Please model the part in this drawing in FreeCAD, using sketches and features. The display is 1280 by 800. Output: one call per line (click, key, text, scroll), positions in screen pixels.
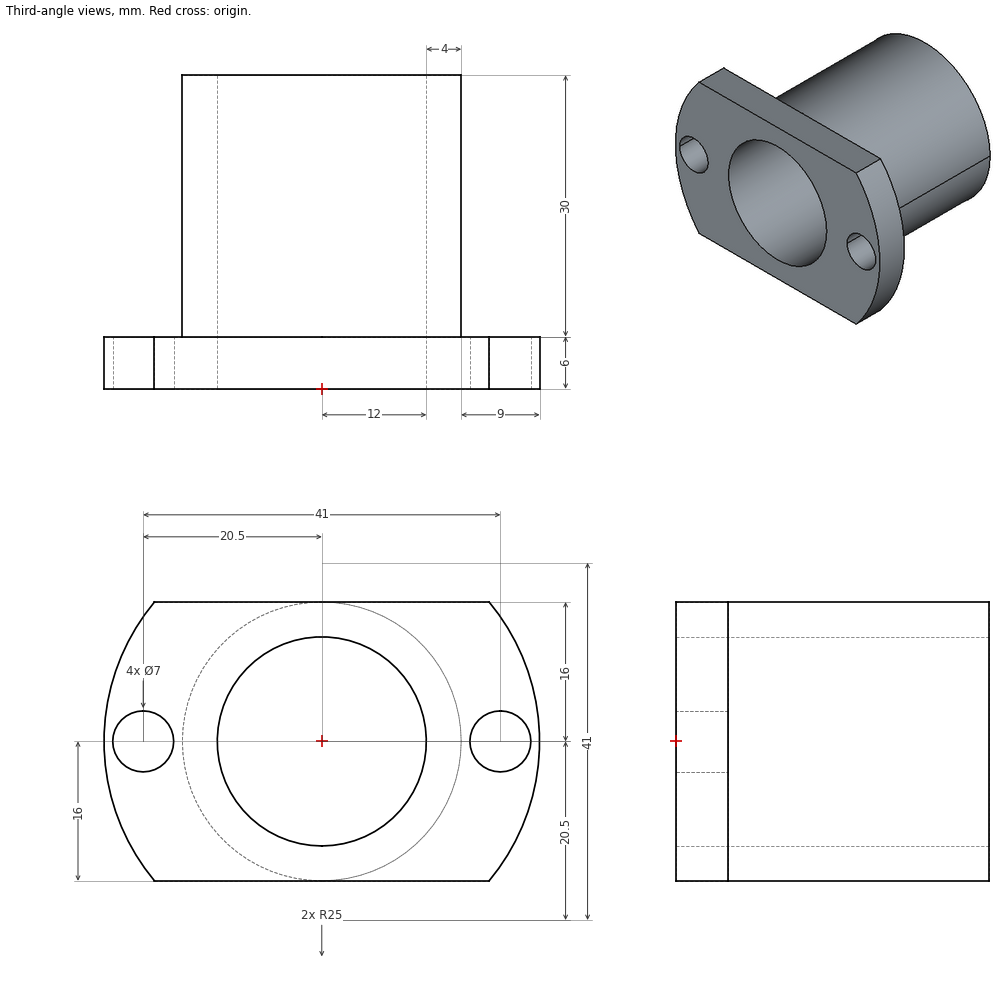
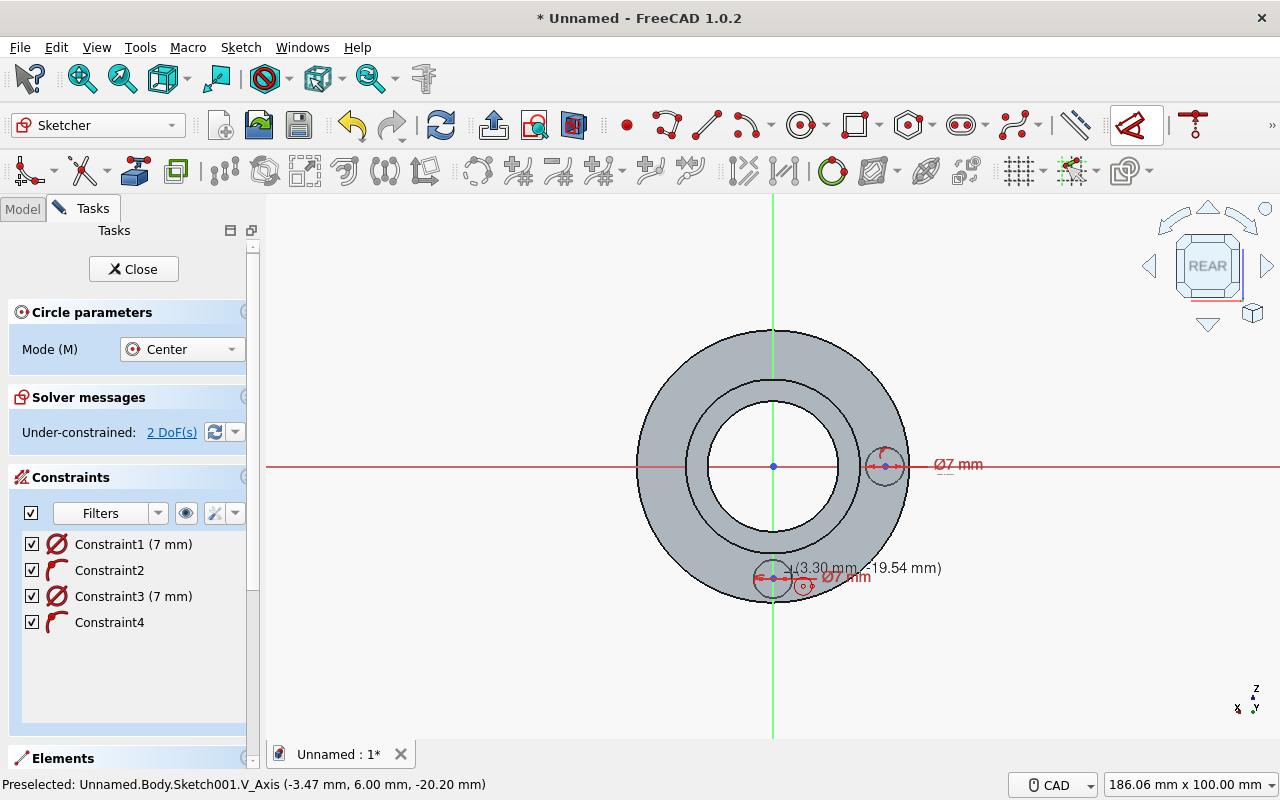
click(661, 466)
move(668, 449)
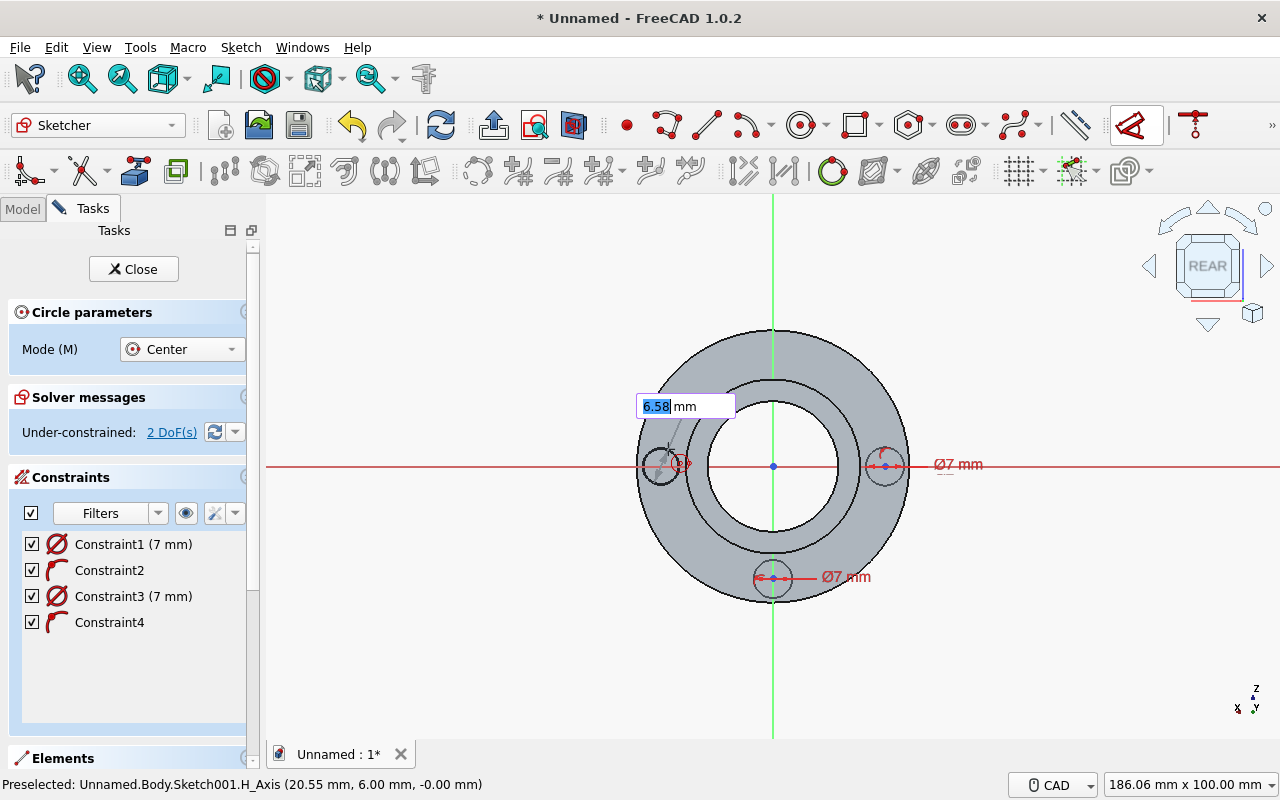
text(7)
key(Return)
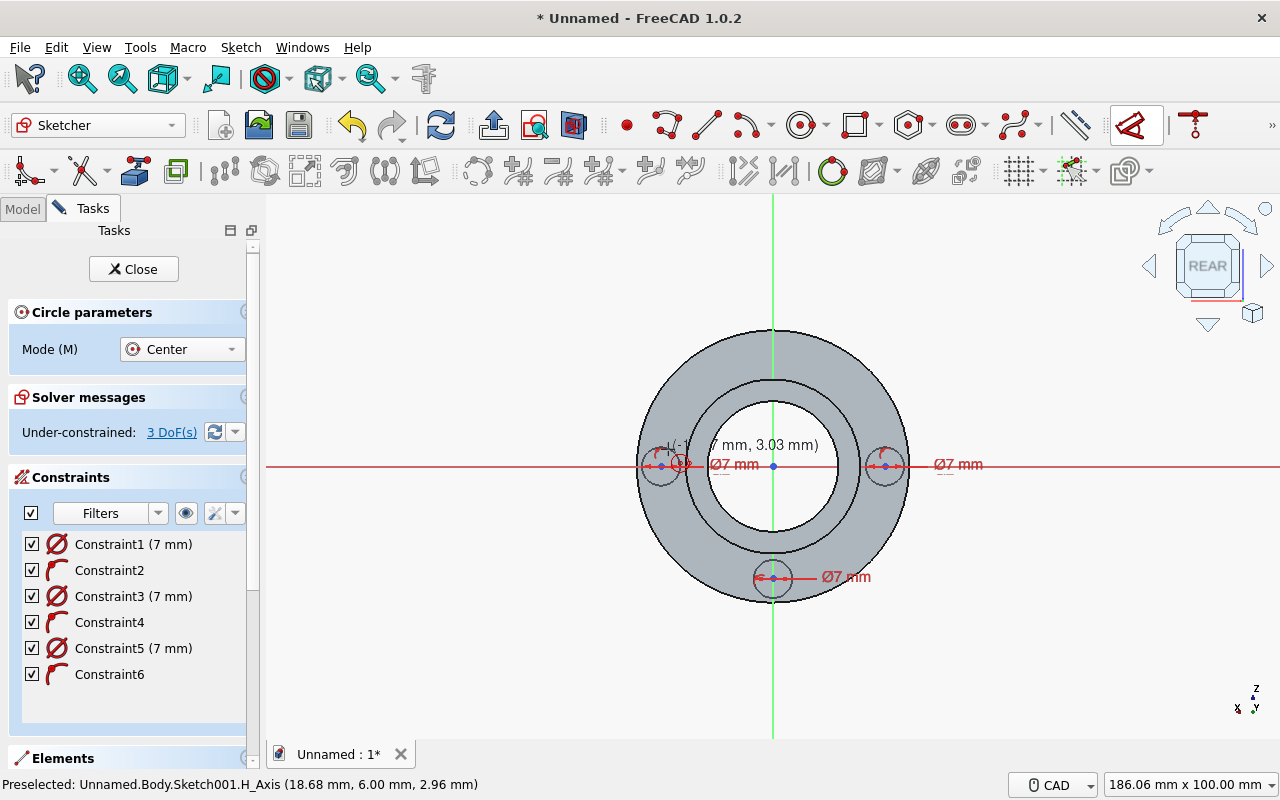
click(773, 355)
move(791, 348)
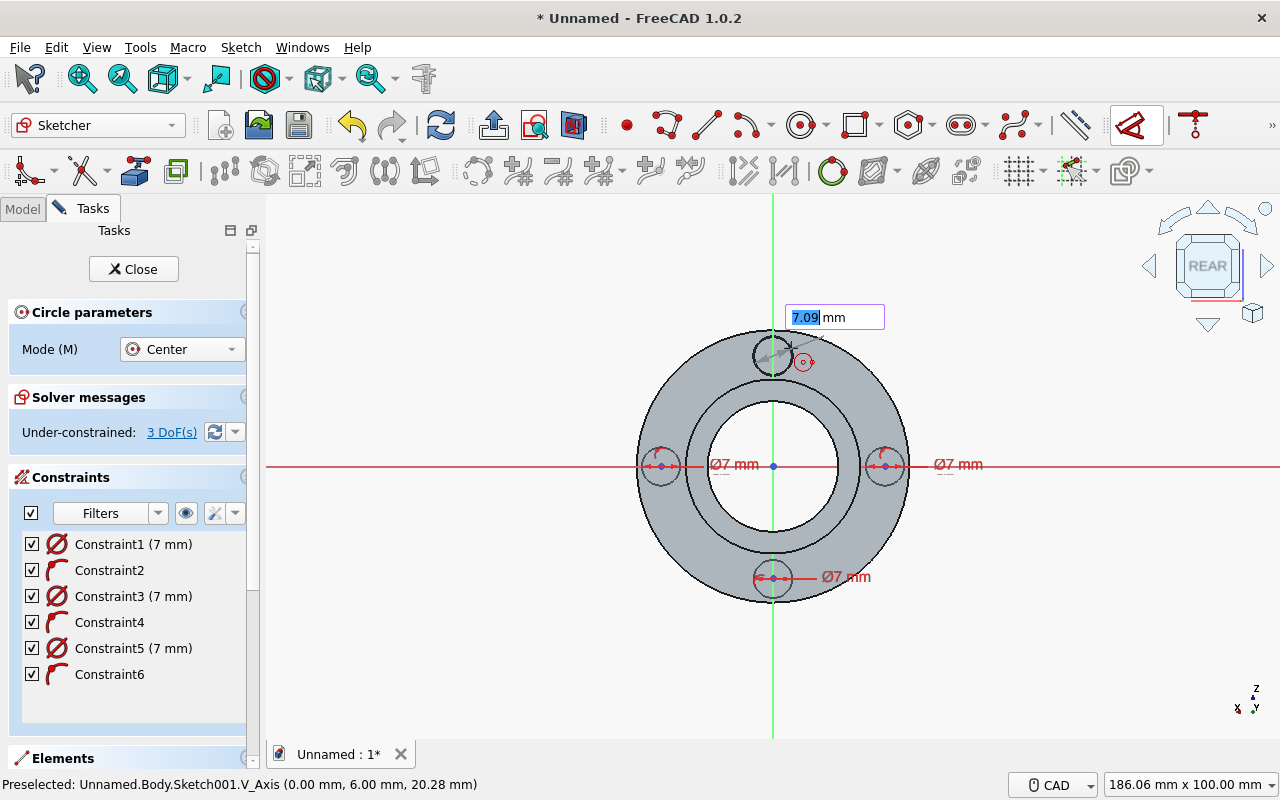
text(7)
key(Return)
key(Escape)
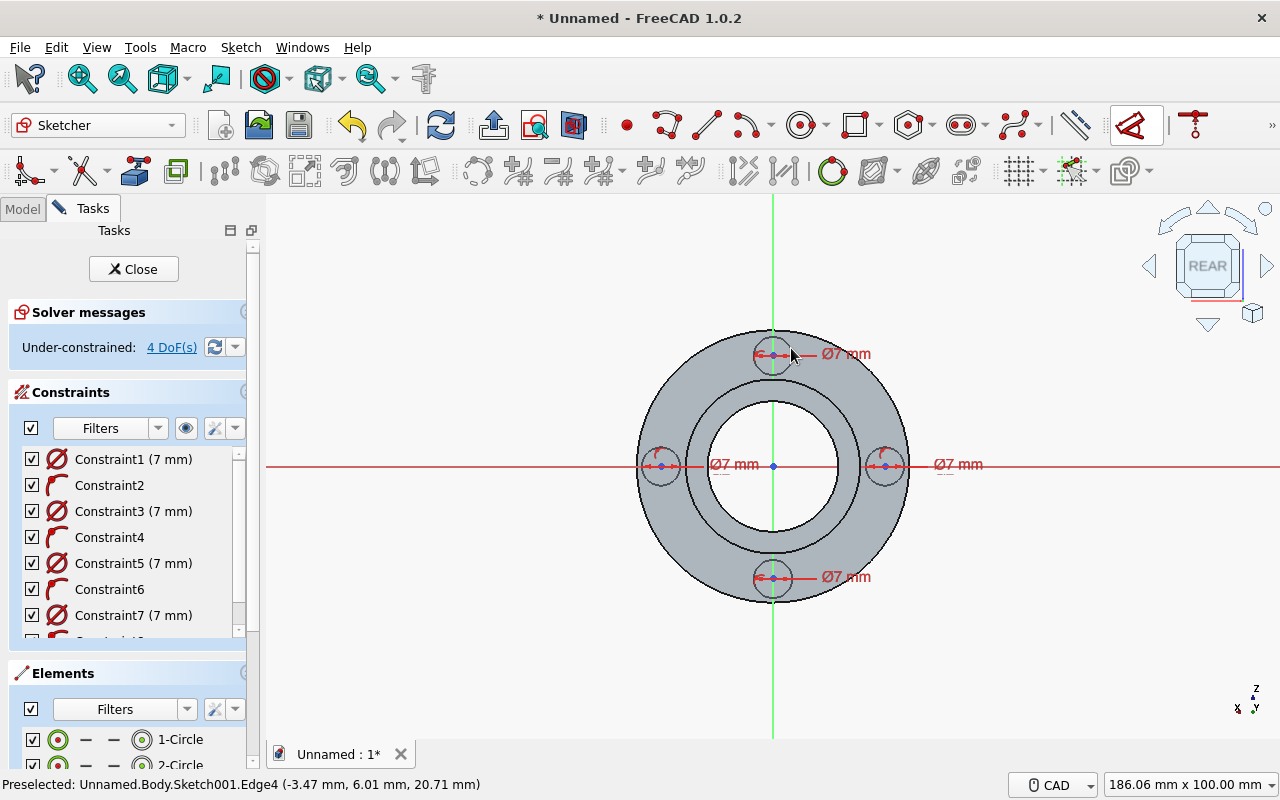
click(885, 466)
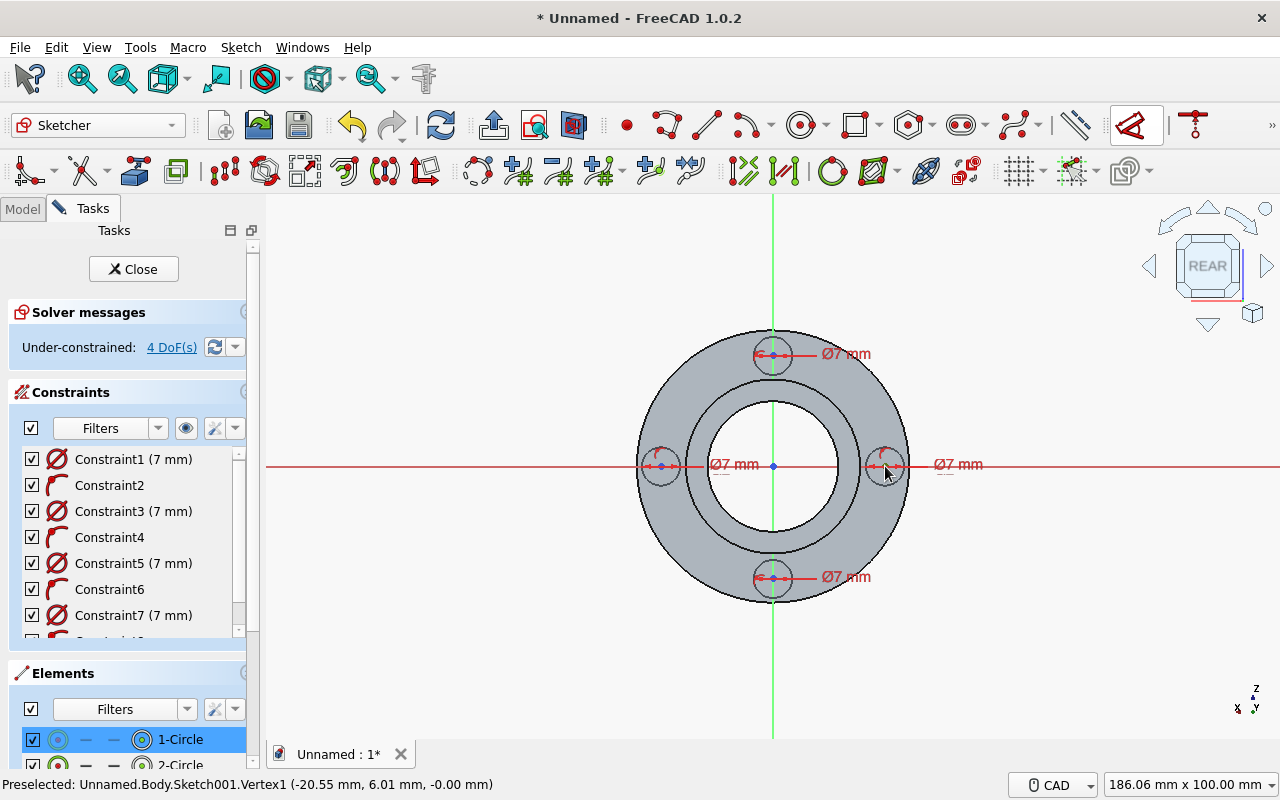
click(661, 466)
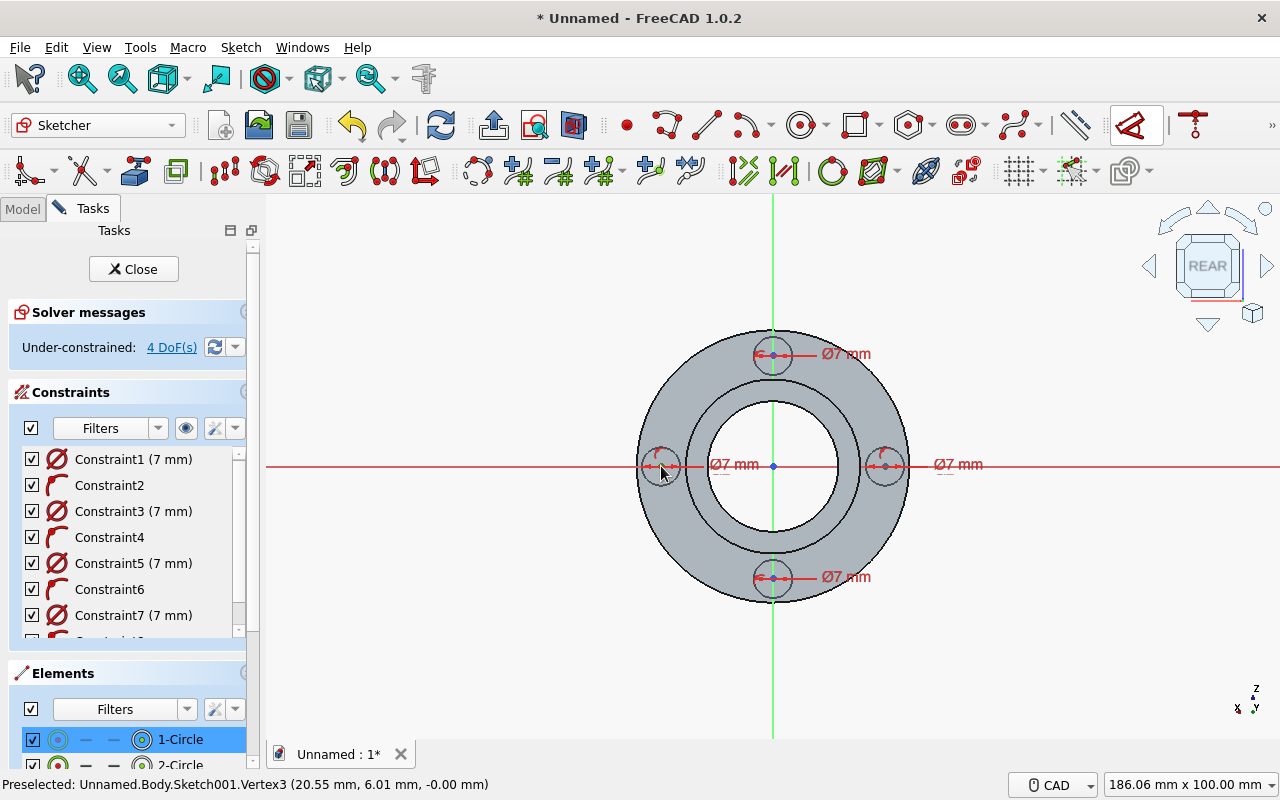
click(1158, 126)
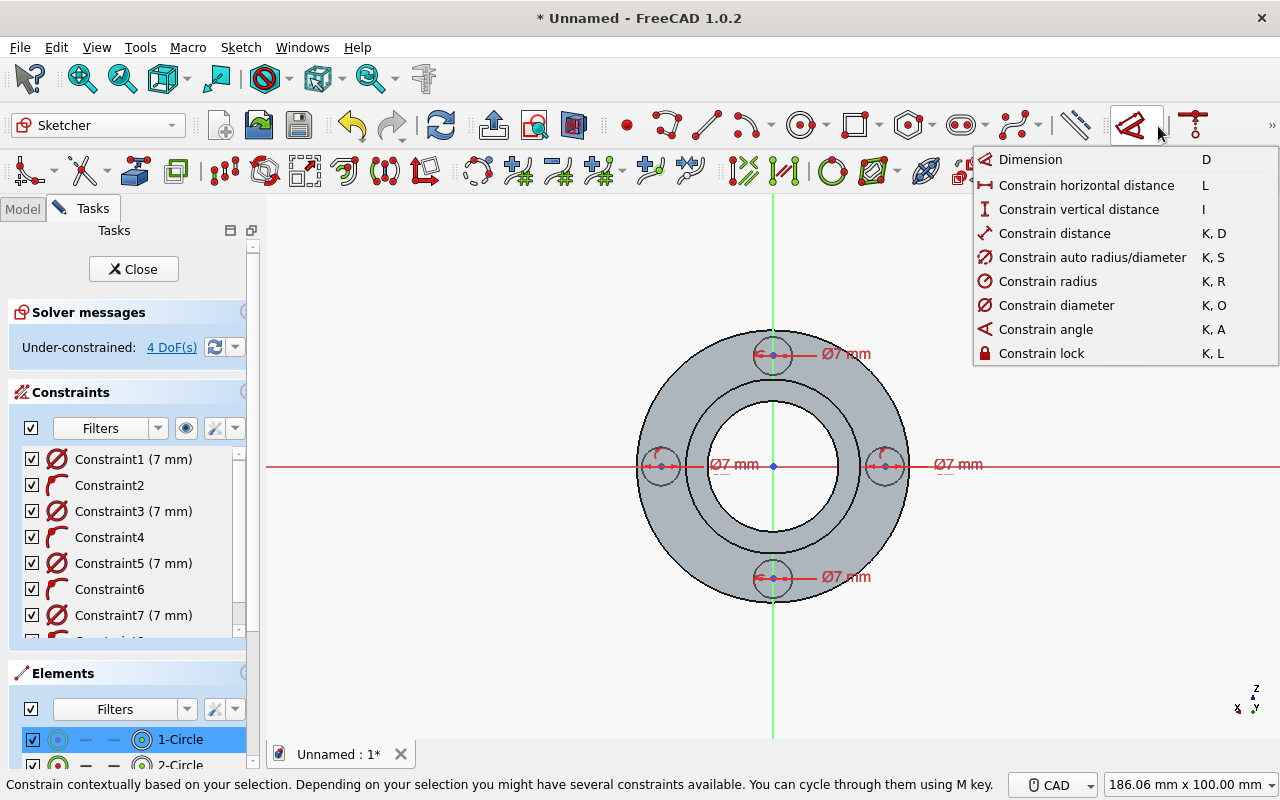
click(1126, 185)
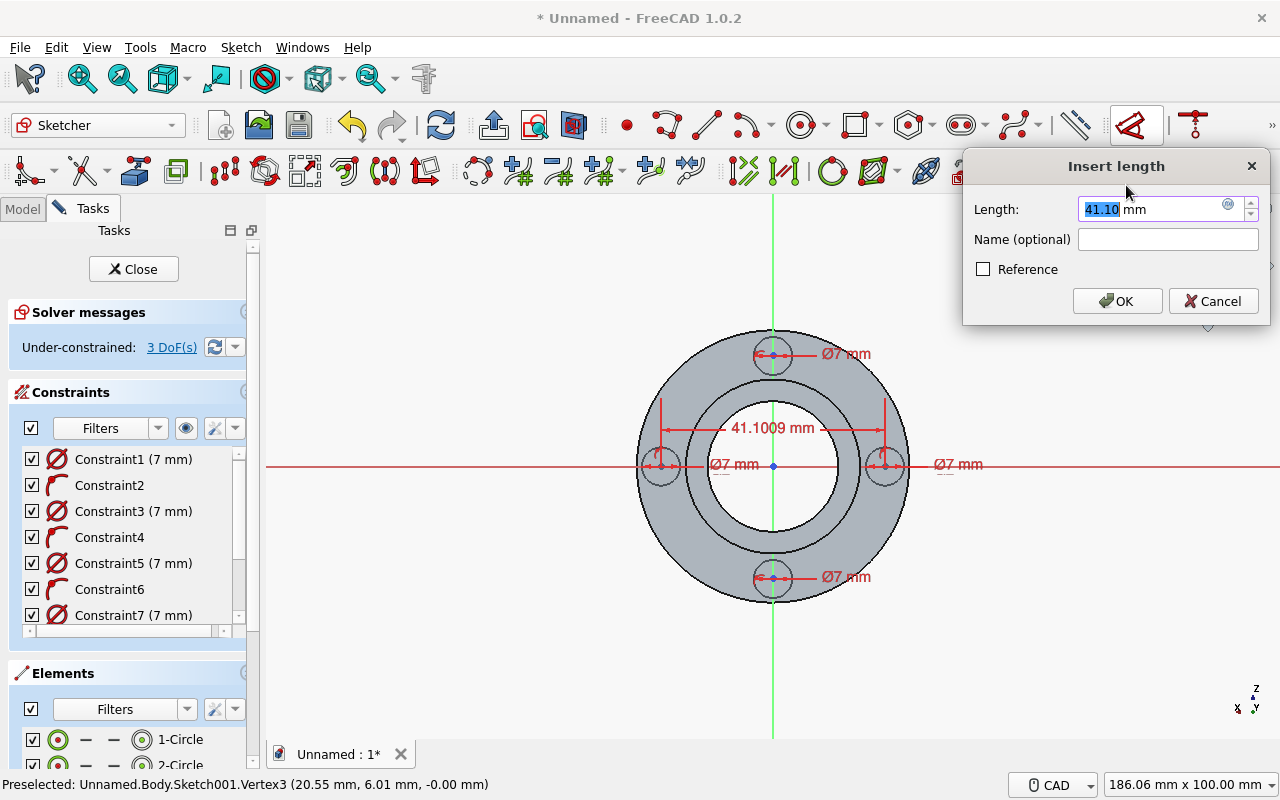
text(41)
key(Return)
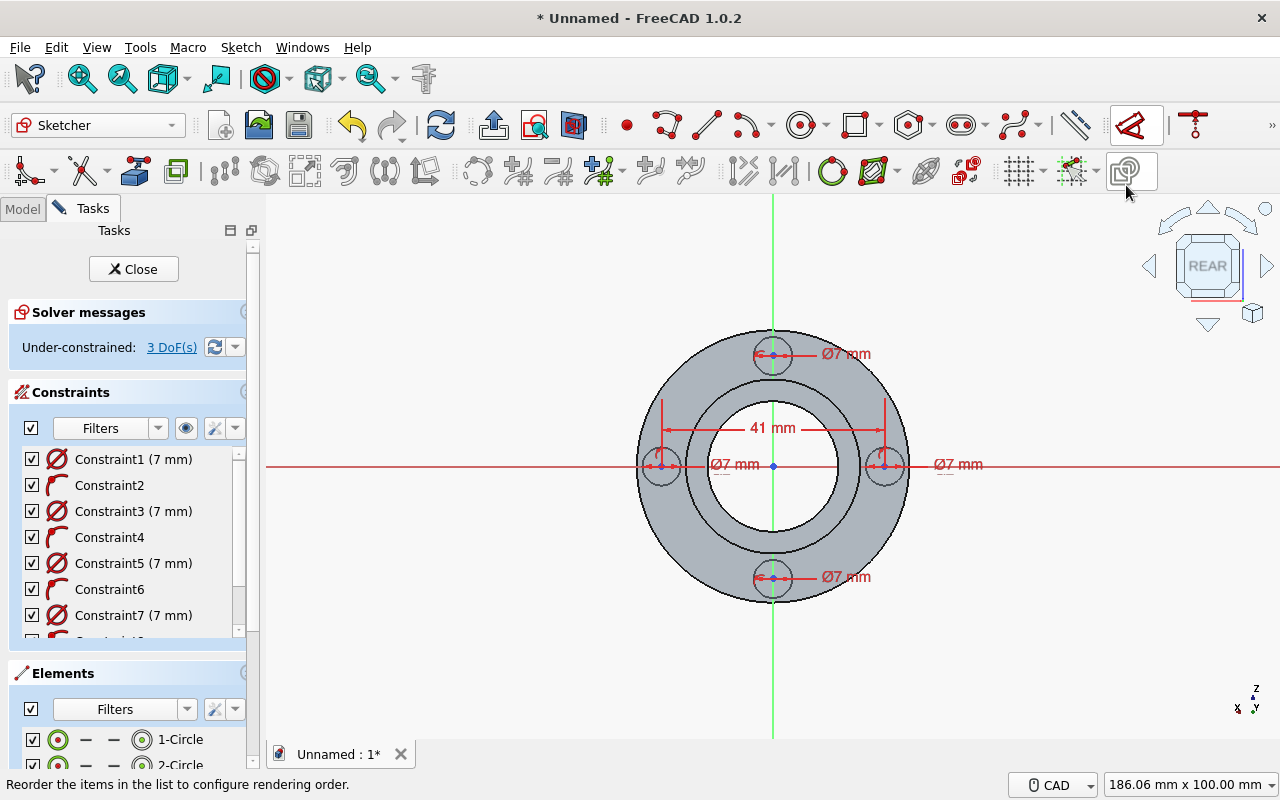
click(773, 579)